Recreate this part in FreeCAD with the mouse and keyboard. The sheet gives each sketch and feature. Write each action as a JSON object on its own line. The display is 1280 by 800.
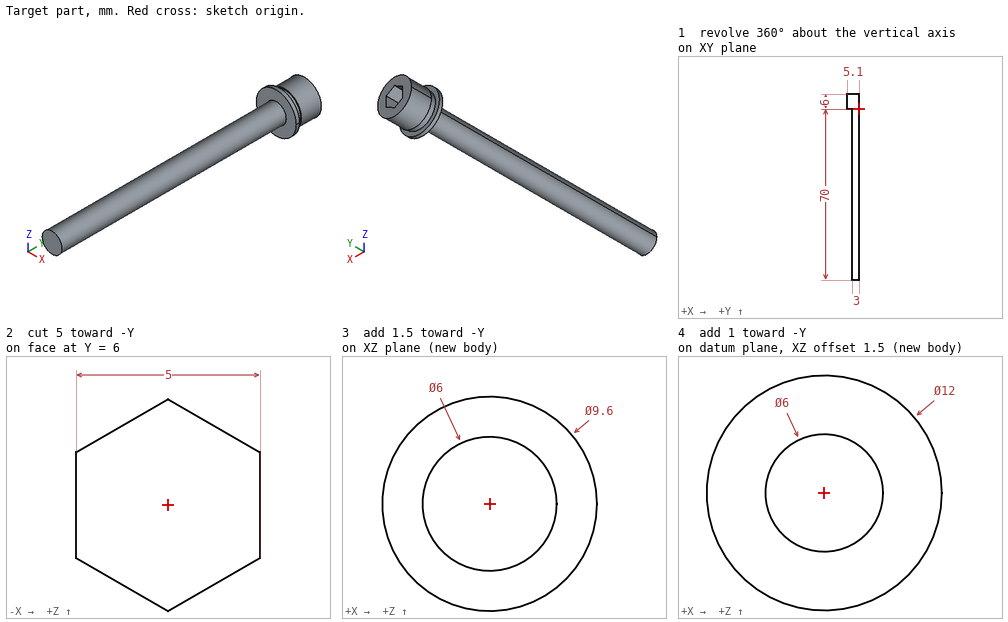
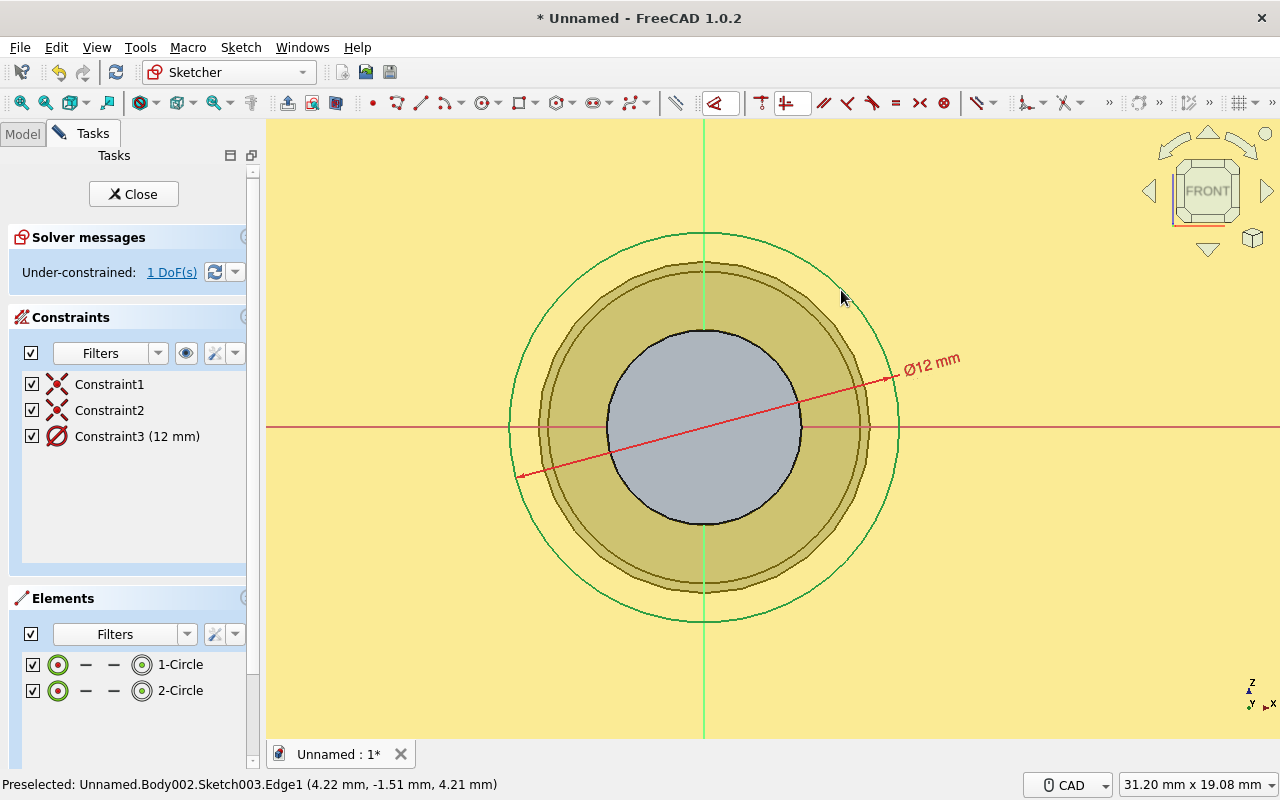
{"action": "left_click", "coordinate": [772, 359]}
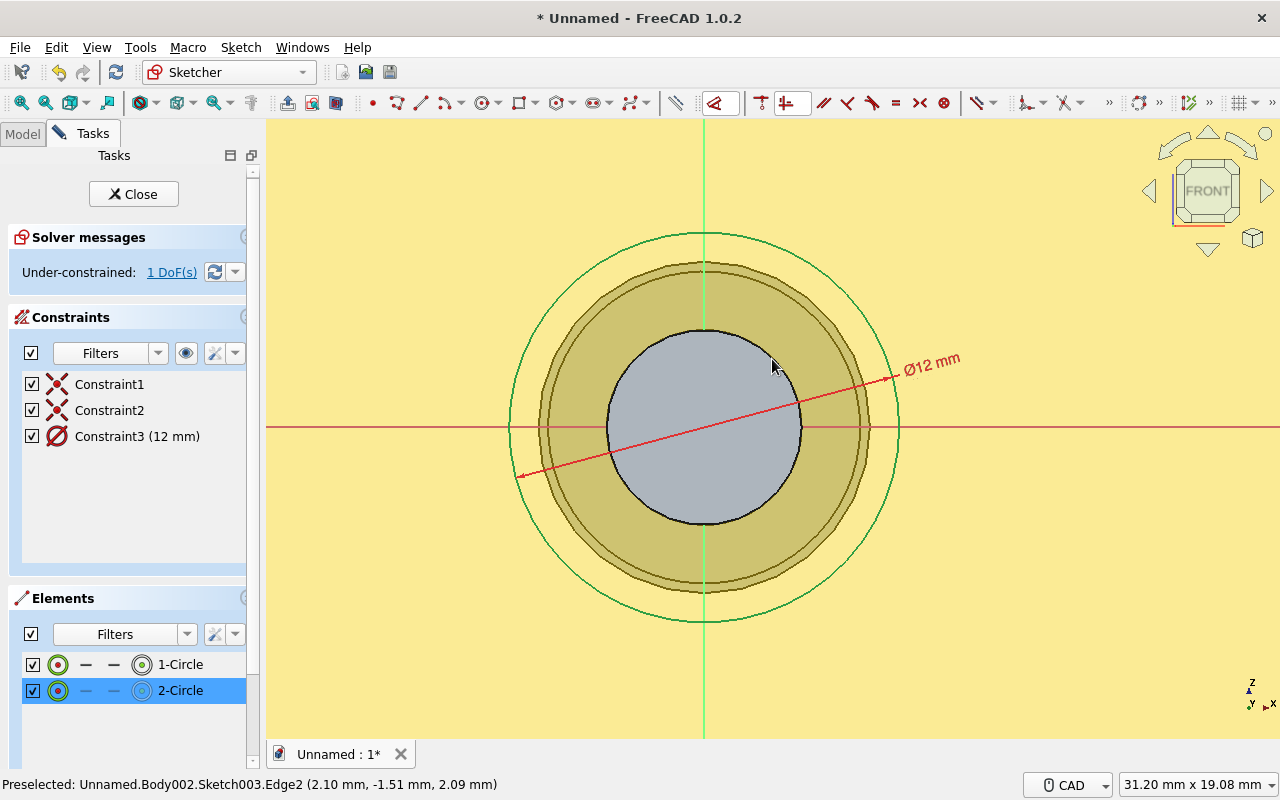
{"action": "key", "text": "k o"}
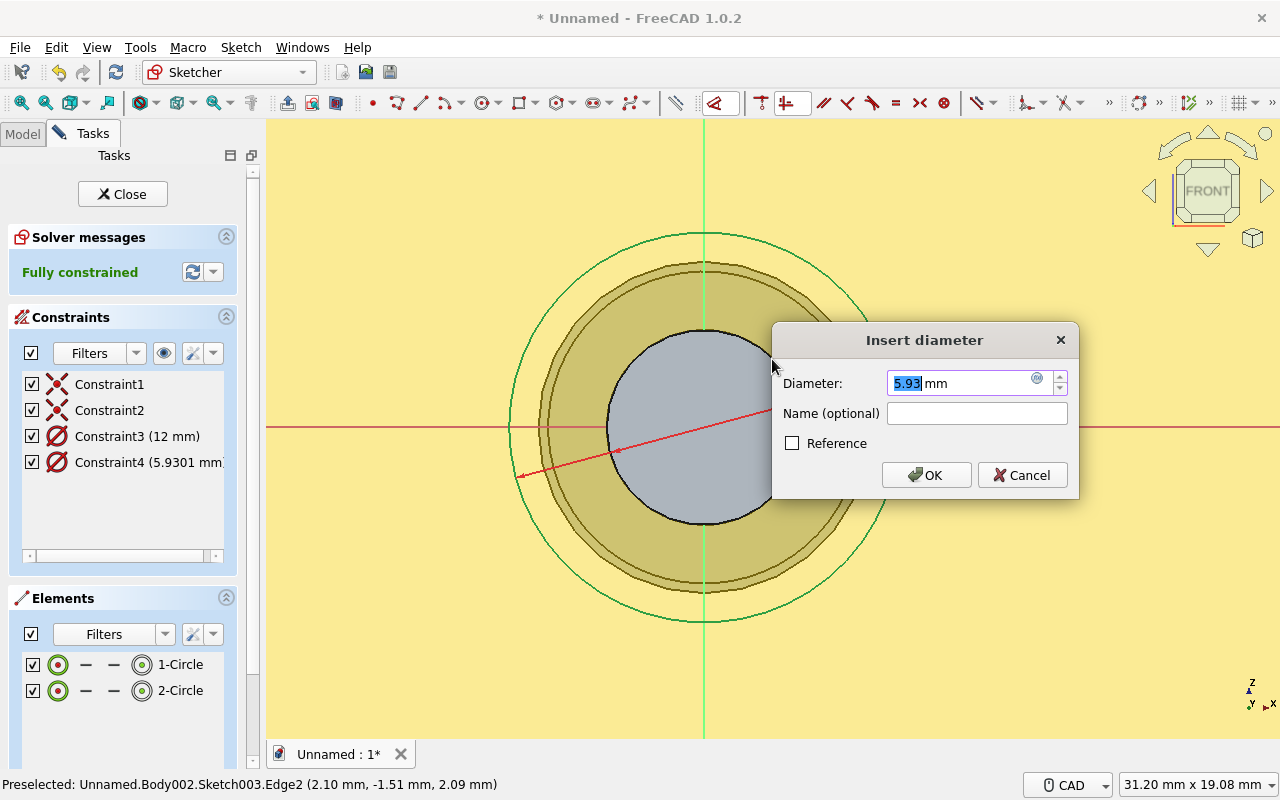
{"action": "type", "text": "6"}
{"action": "key", "text": "Return"}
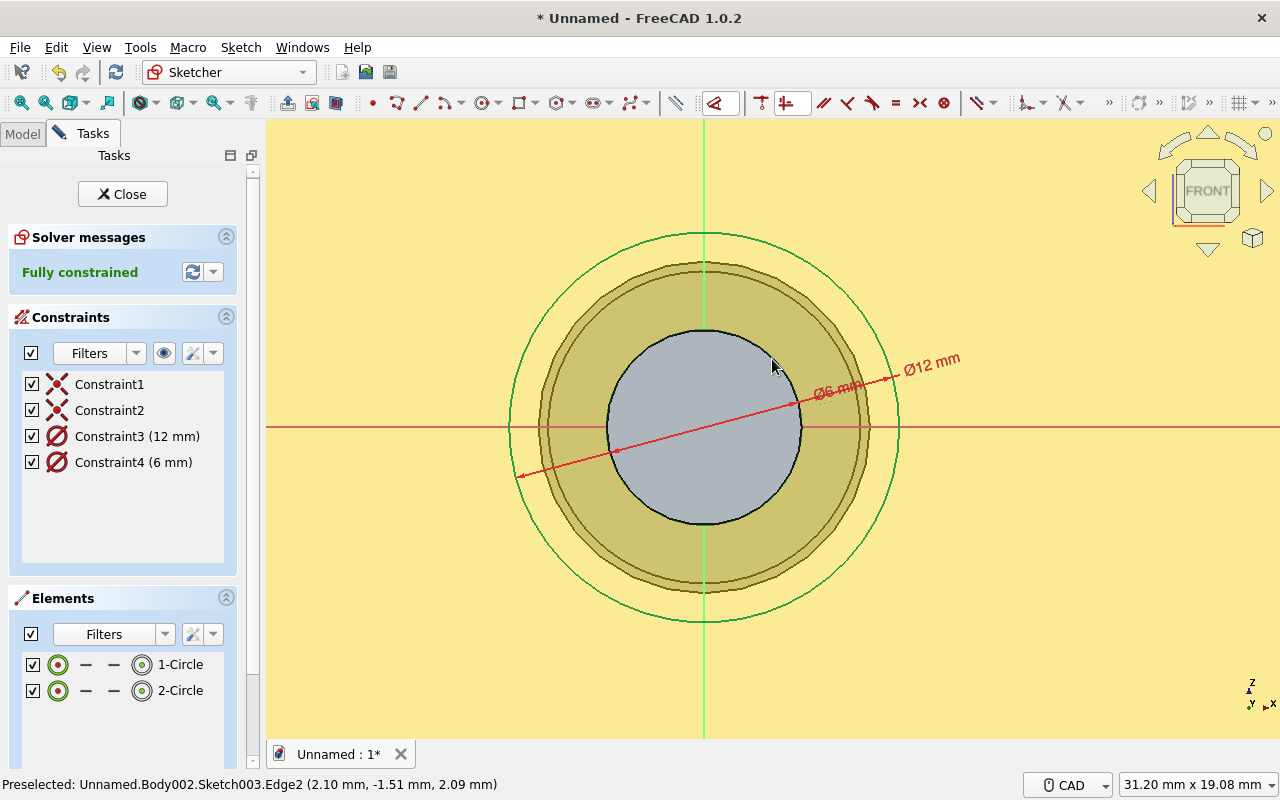
{"action": "left_click", "coordinate": [123, 194]}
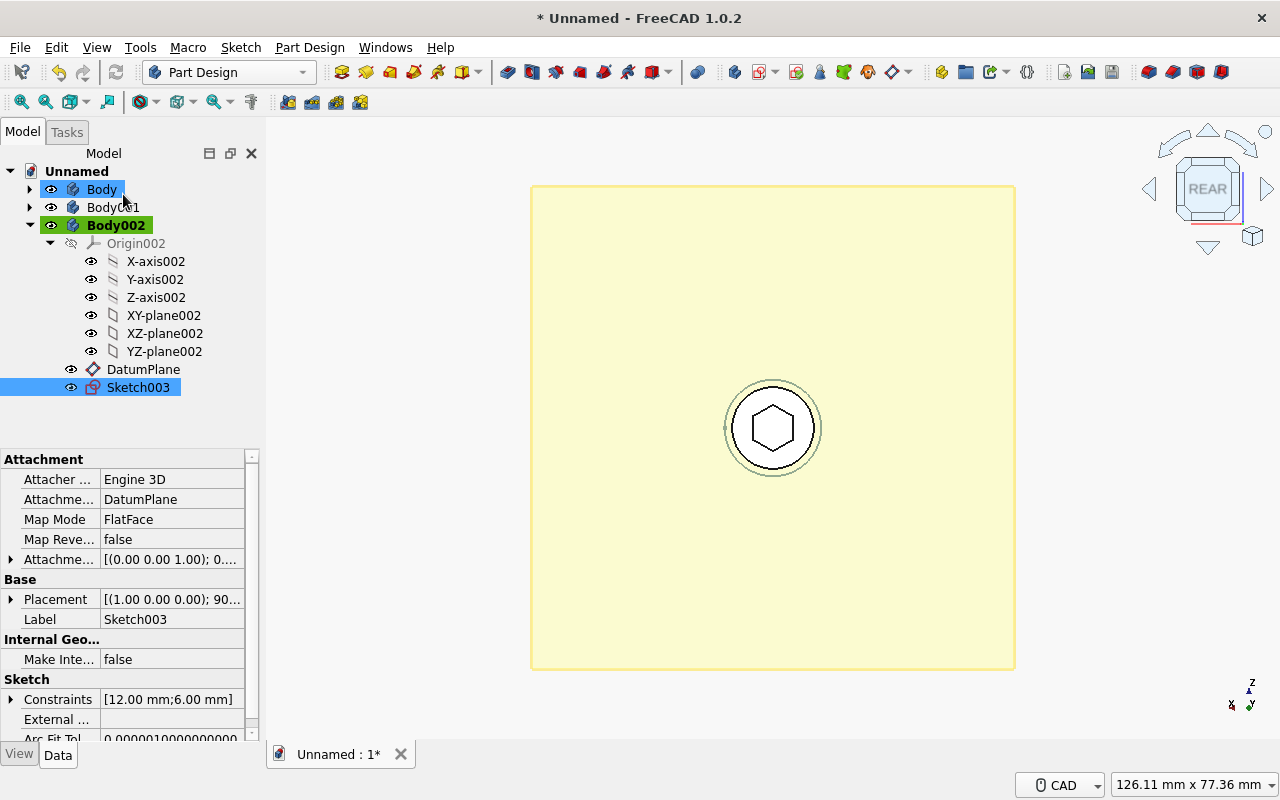
{"action": "left_click", "coordinate": [342, 72]}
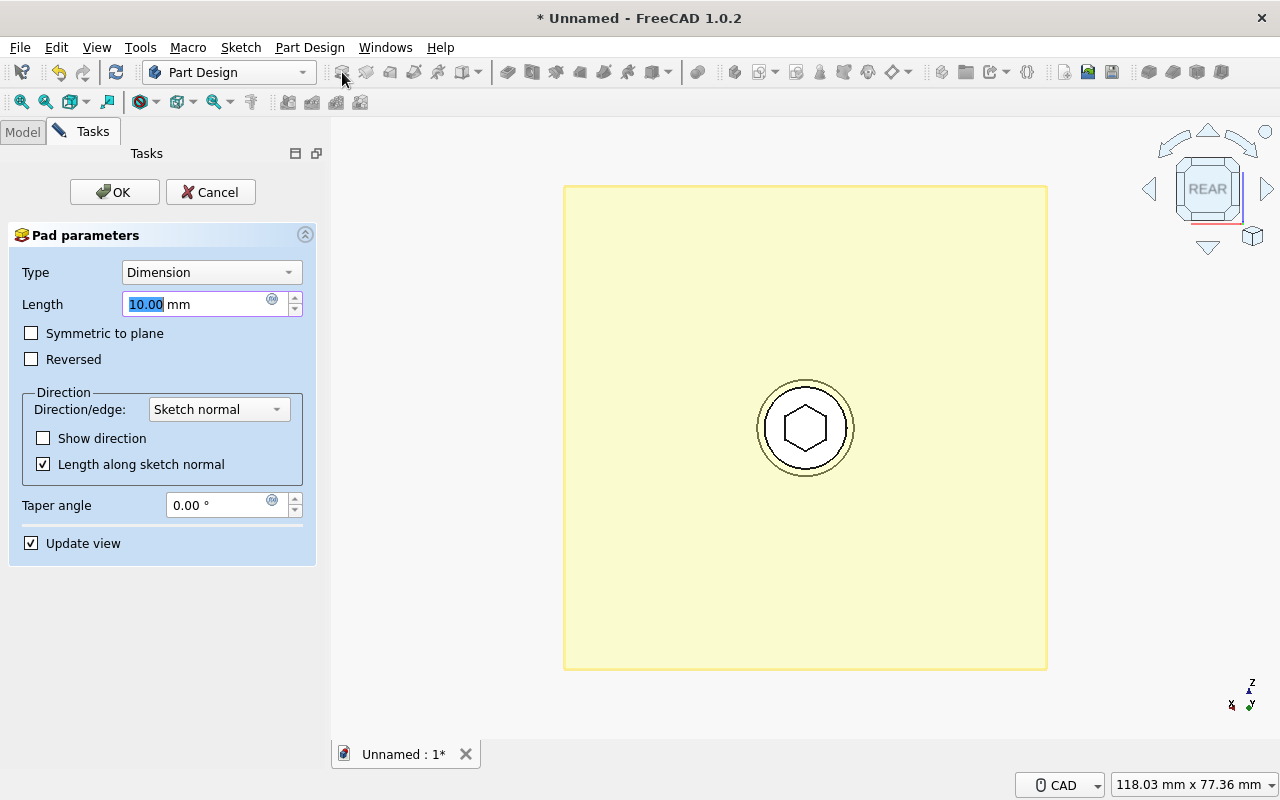
{"action": "type", "text": "1"}
{"action": "key", "text": "Tab"}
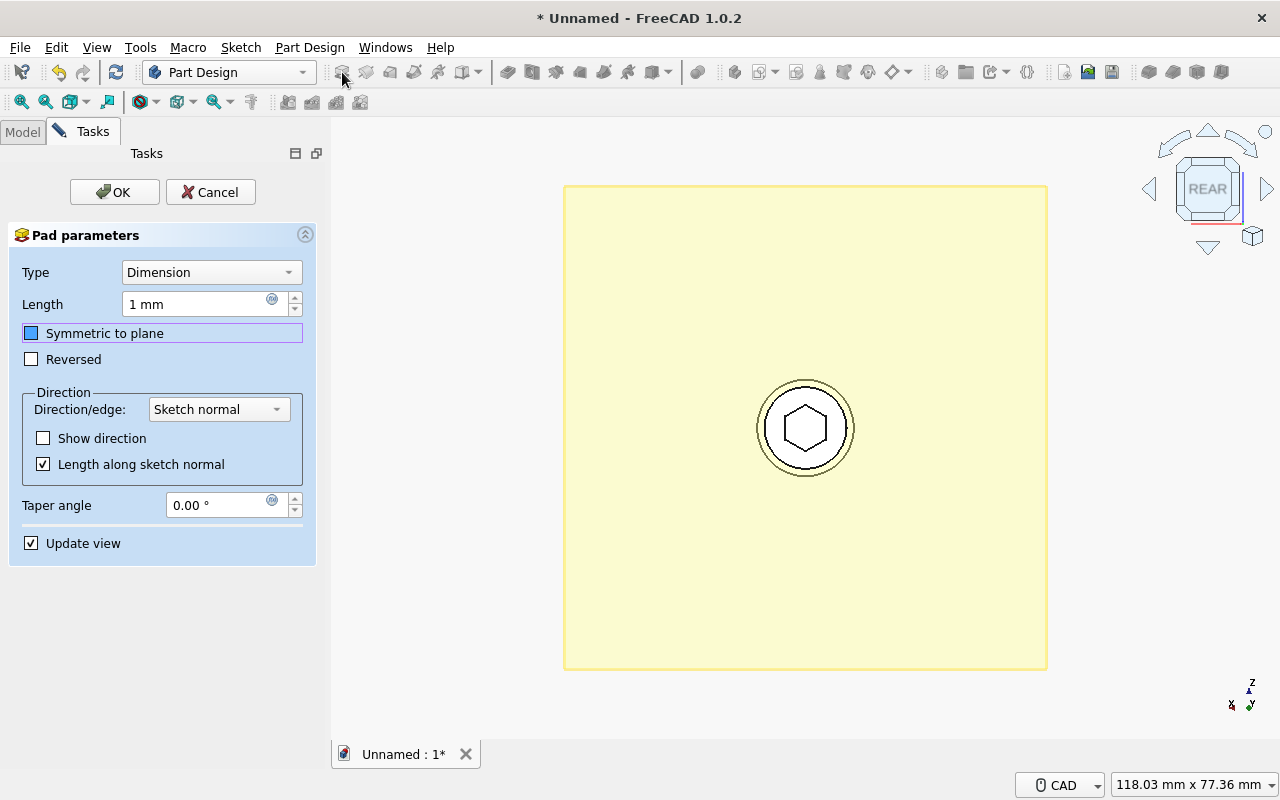
{"action": "left_click", "coordinate": [115, 192]}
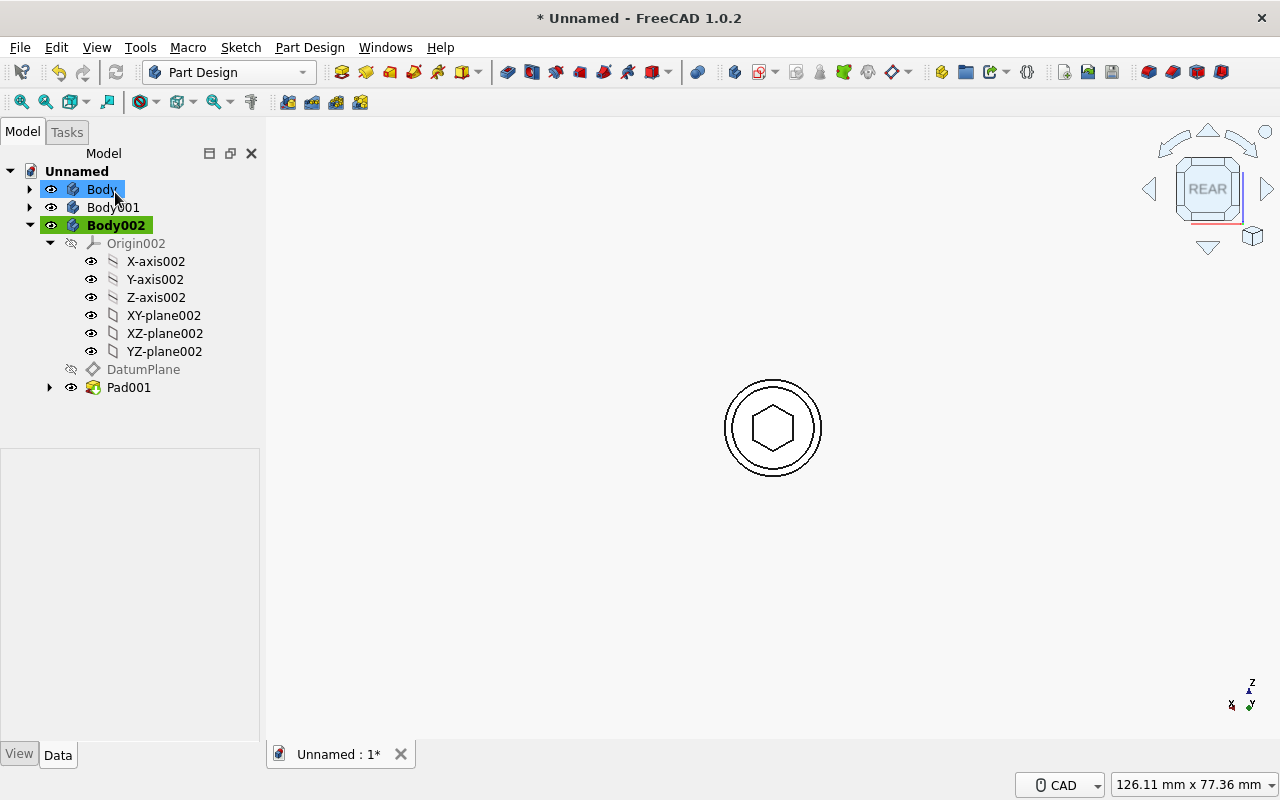
{"action": "key", "text": "0"}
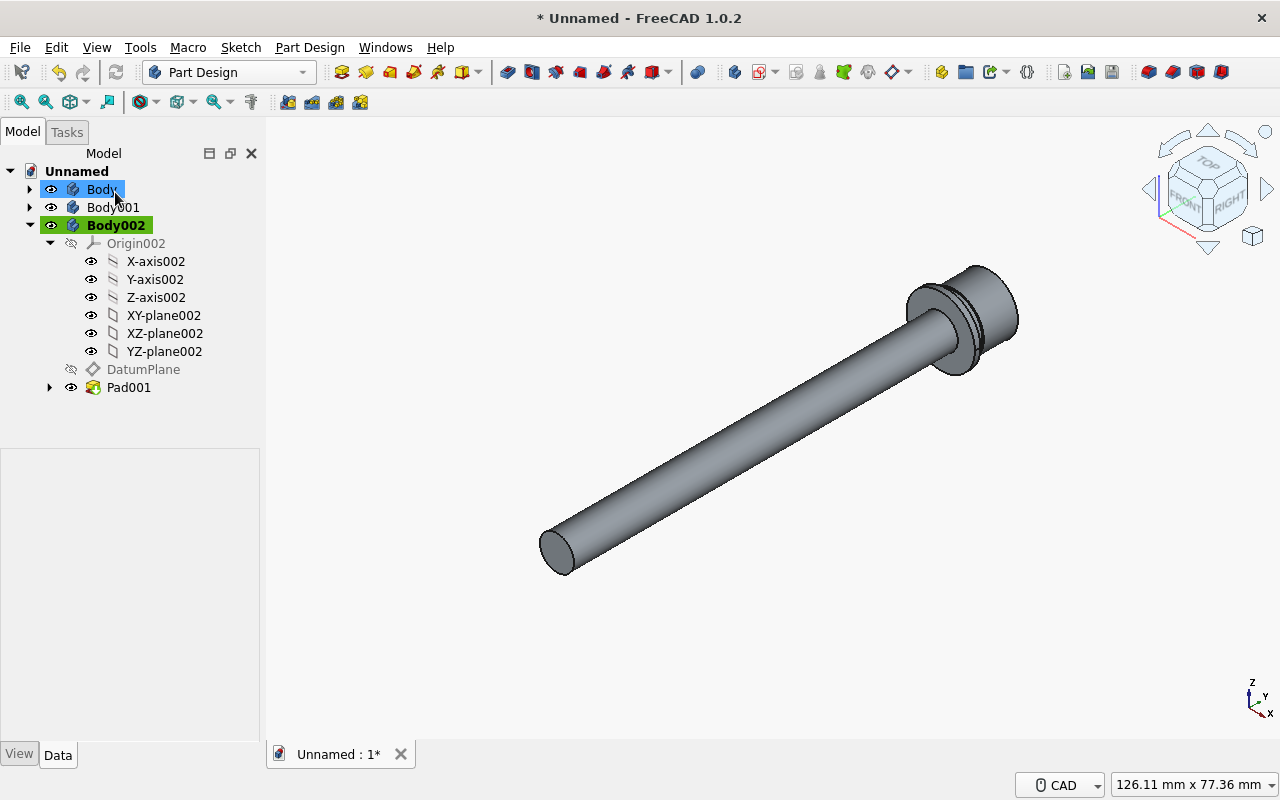
{"action": "key", "text": "v f"}